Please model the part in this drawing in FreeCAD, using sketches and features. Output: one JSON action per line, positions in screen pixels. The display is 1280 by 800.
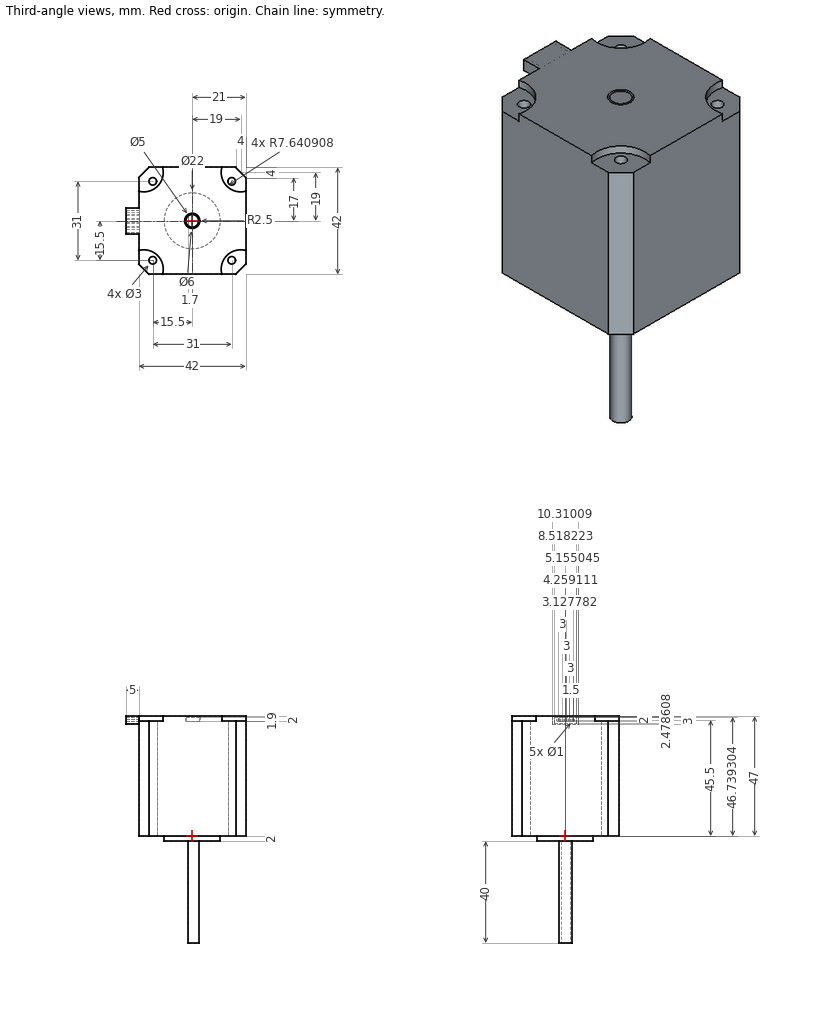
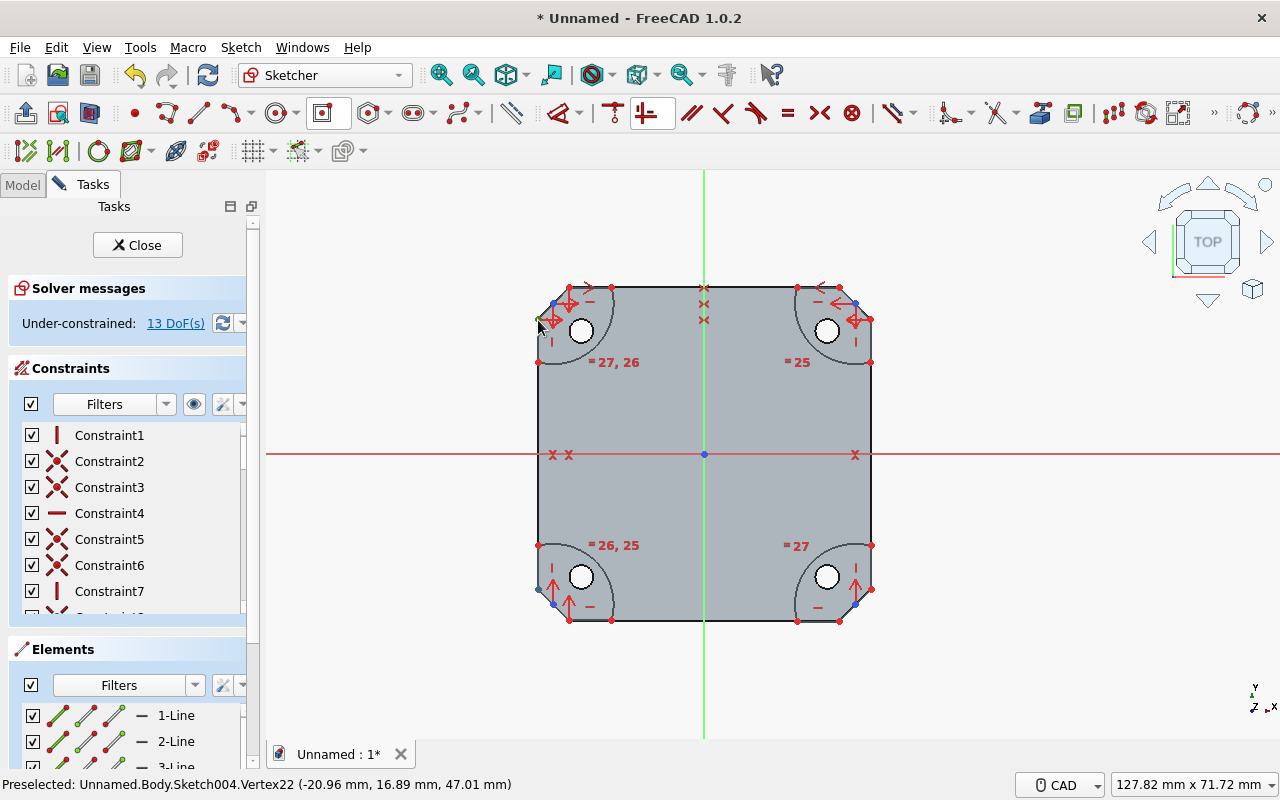
{"action": "left_click", "coordinate": [353, 454]}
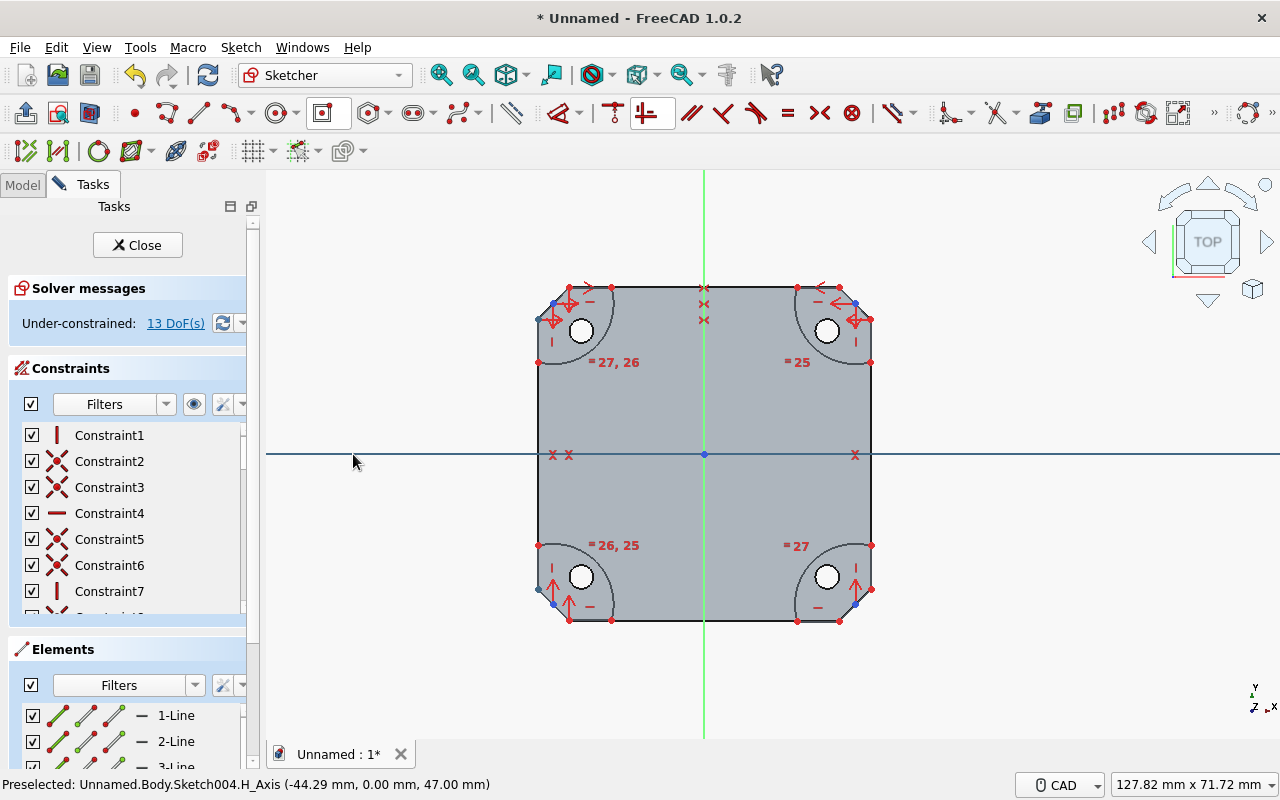
{"action": "left_click", "coordinate": [820, 114]}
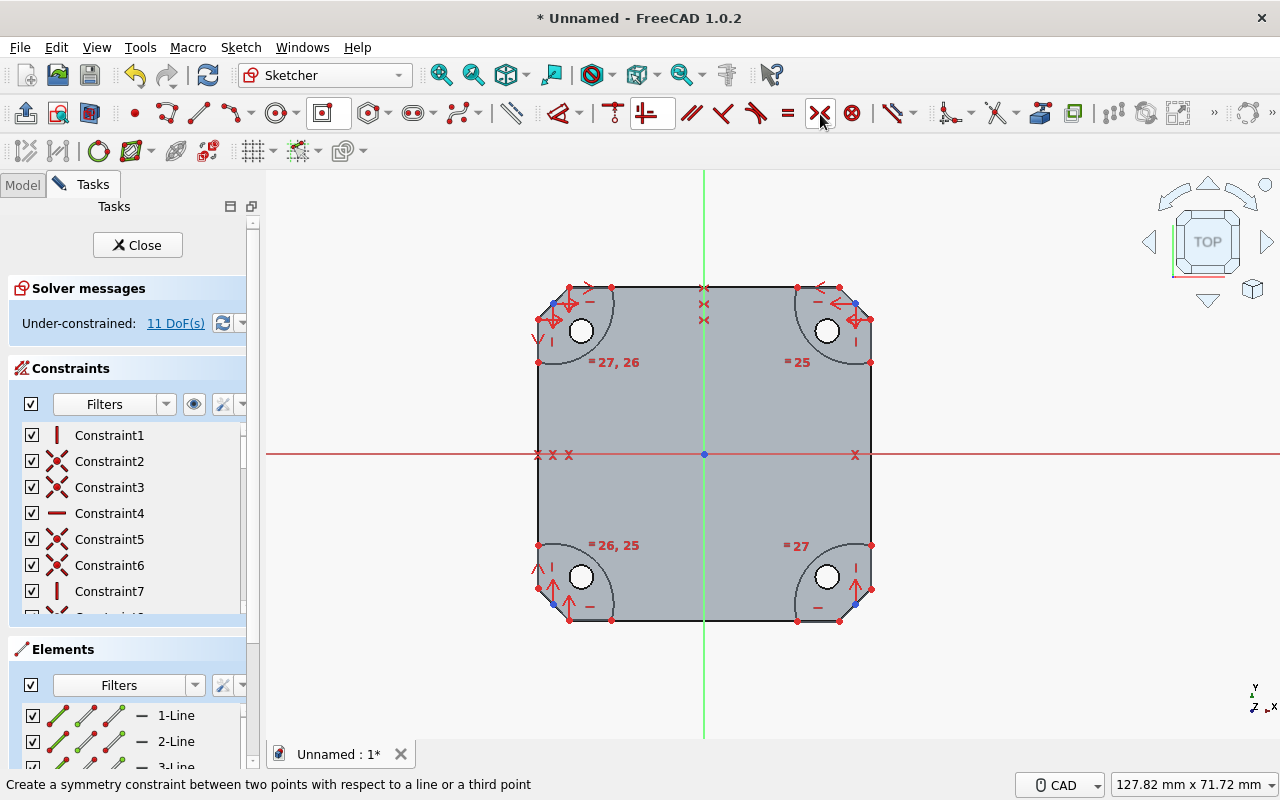
{"action": "left_click", "coordinate": [840, 288]}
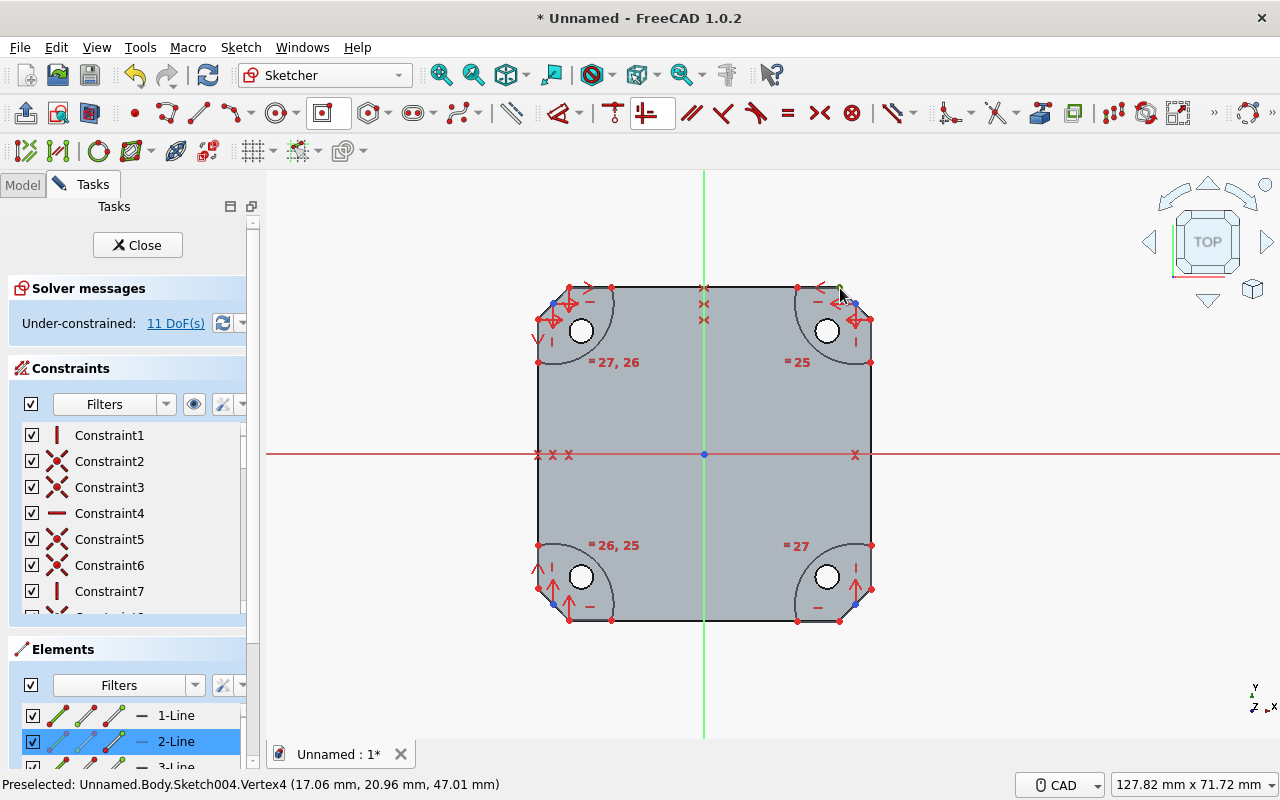
{"action": "left_click", "coordinate": [839, 622]}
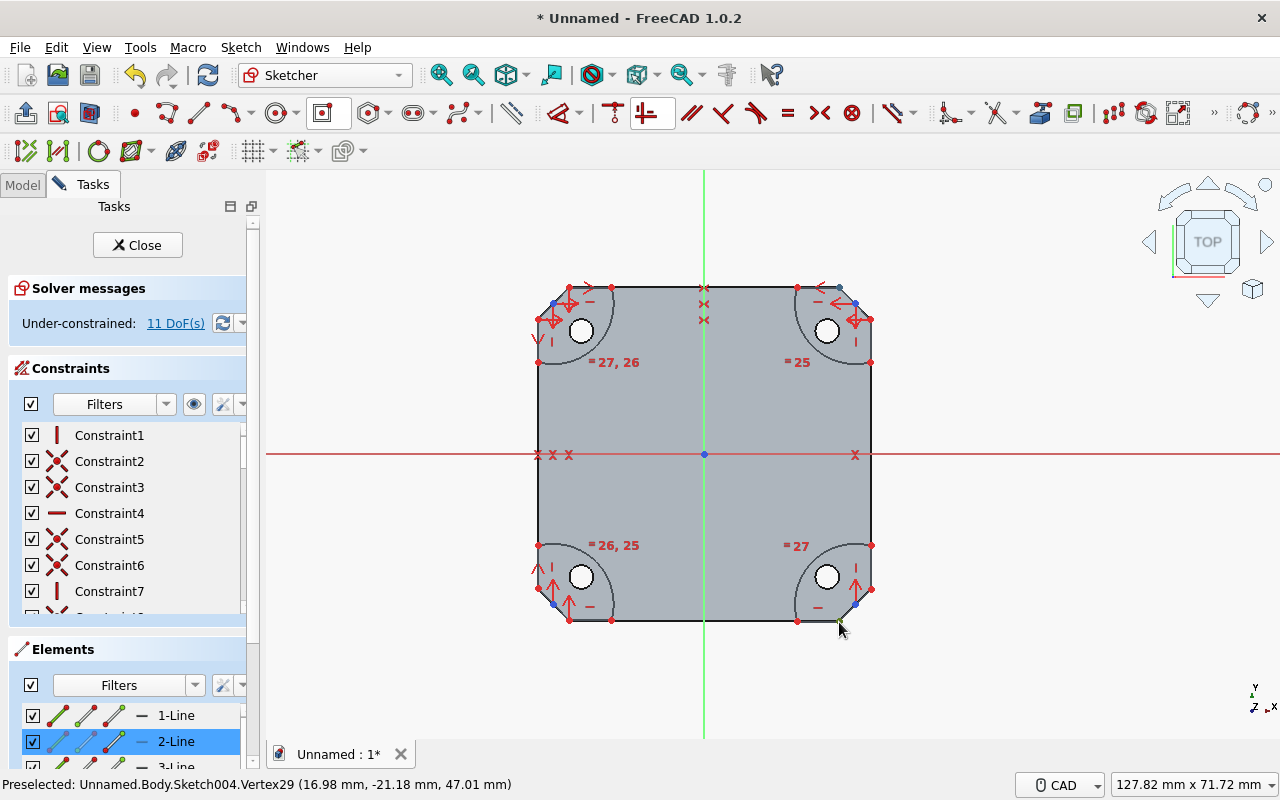
{"action": "left_click", "coordinate": [353, 454]}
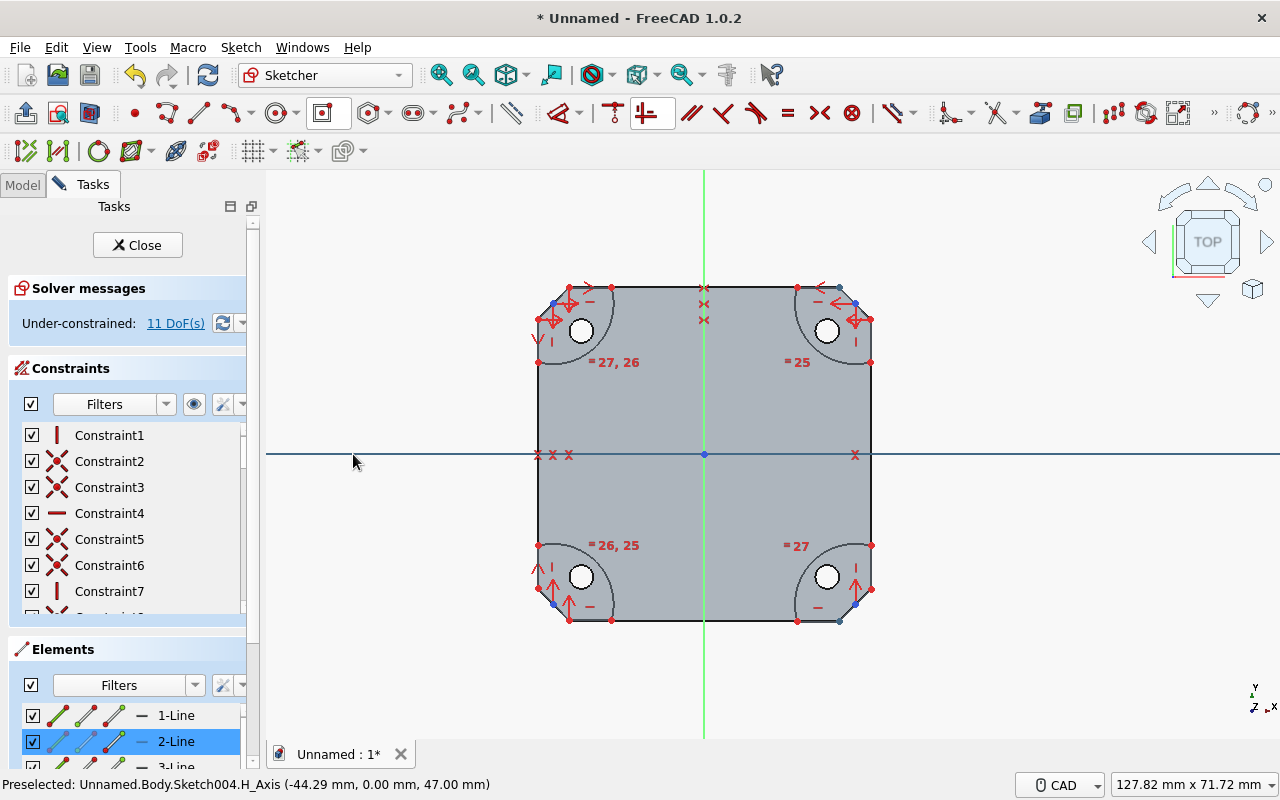
{"action": "key", "text": "s"}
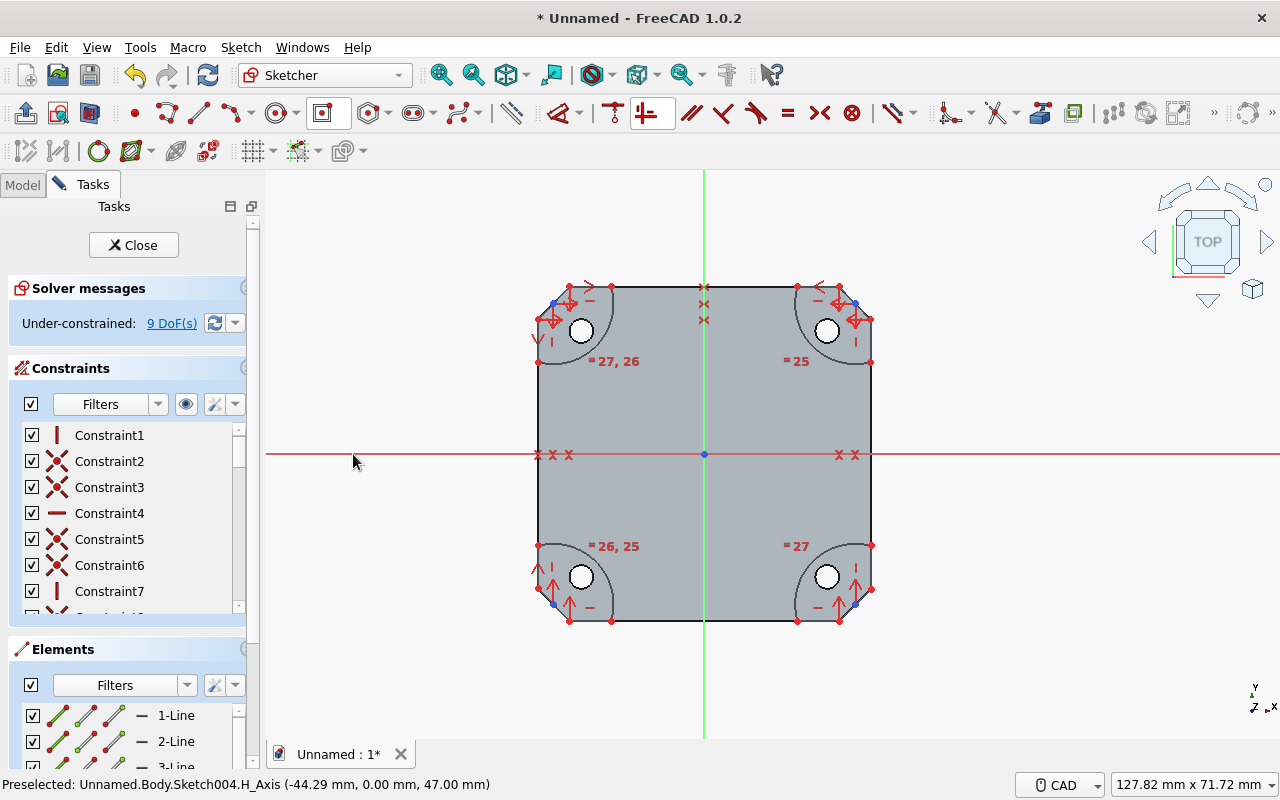
{"action": "left_click", "coordinate": [871, 320]}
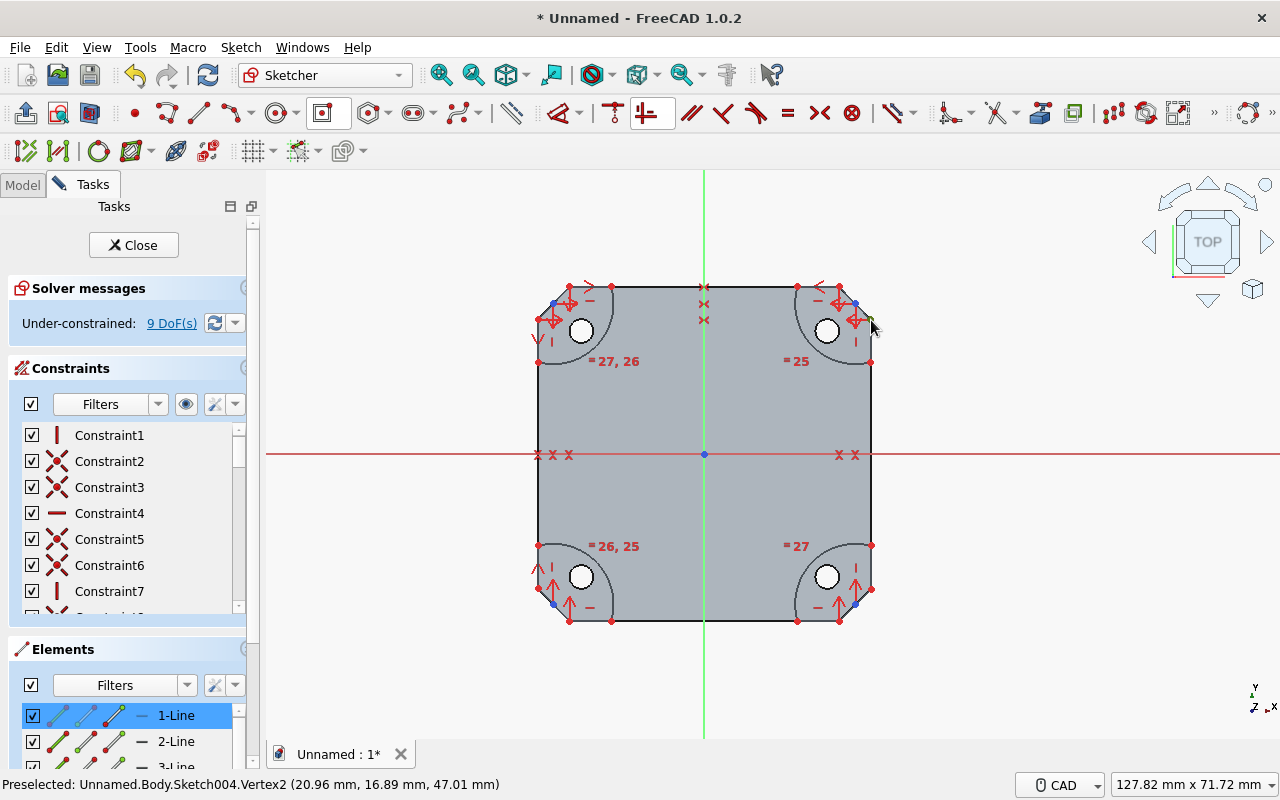
{"action": "left_click", "coordinate": [871, 590]}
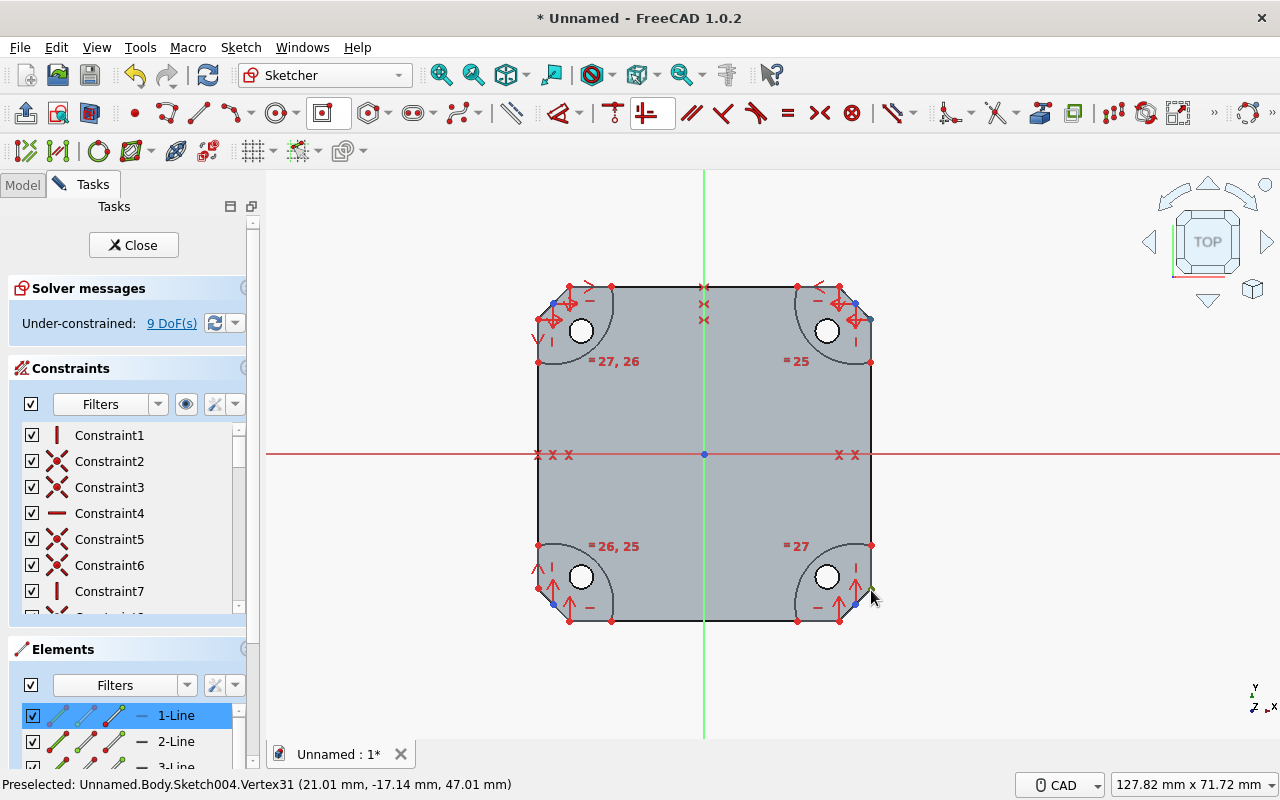
{"action": "left_click", "coordinate": [353, 454]}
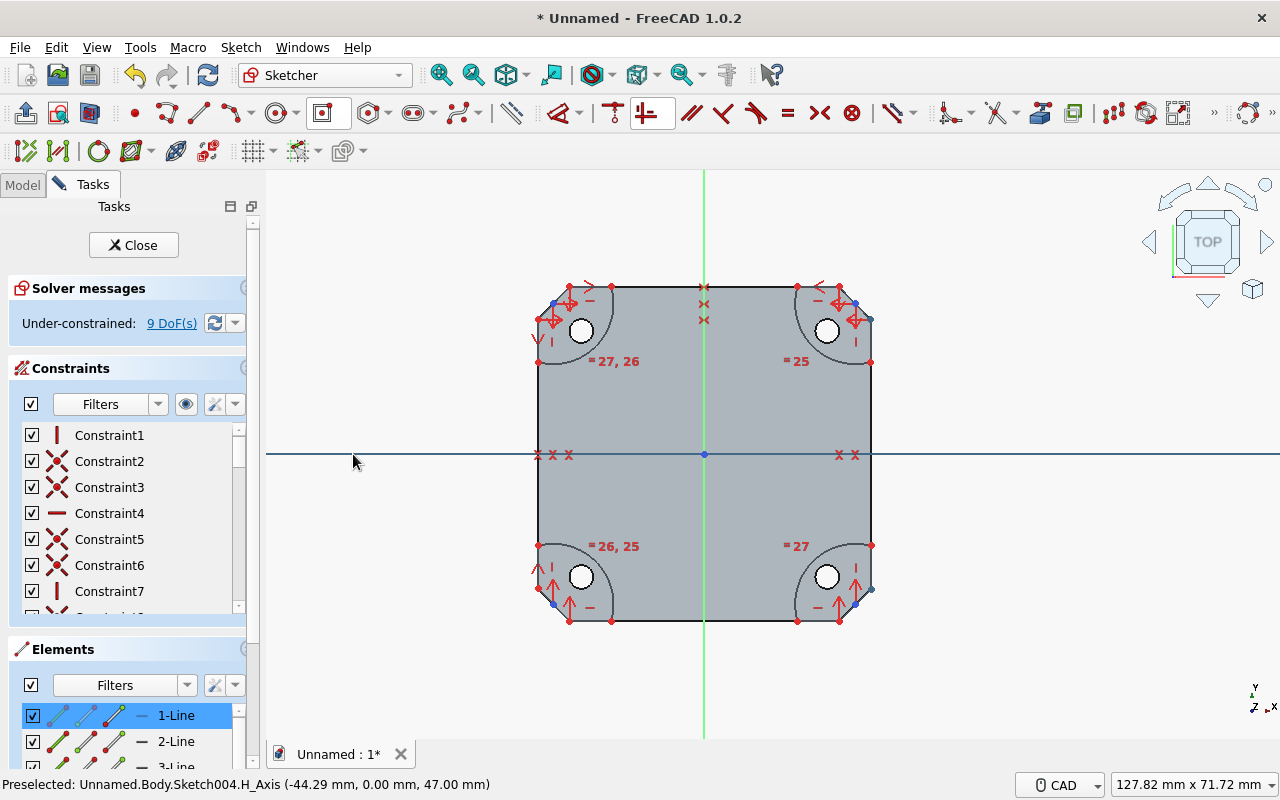
{"action": "left_click", "coordinate": [820, 114]}